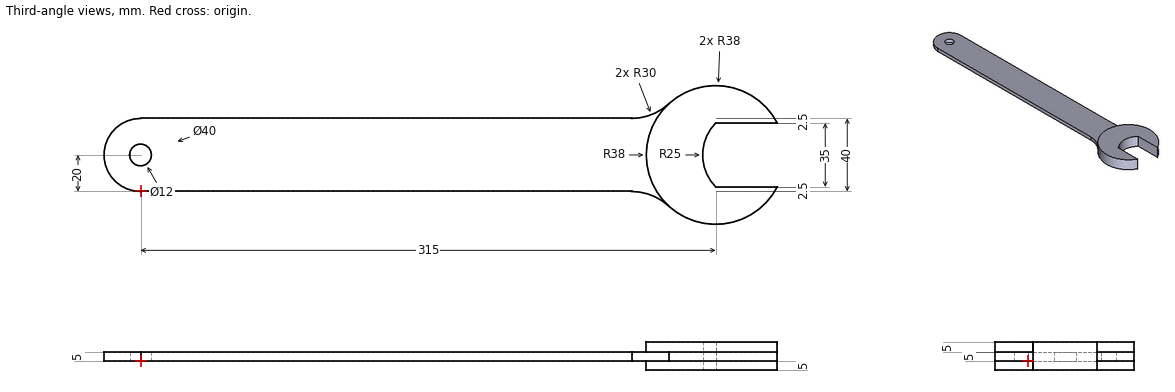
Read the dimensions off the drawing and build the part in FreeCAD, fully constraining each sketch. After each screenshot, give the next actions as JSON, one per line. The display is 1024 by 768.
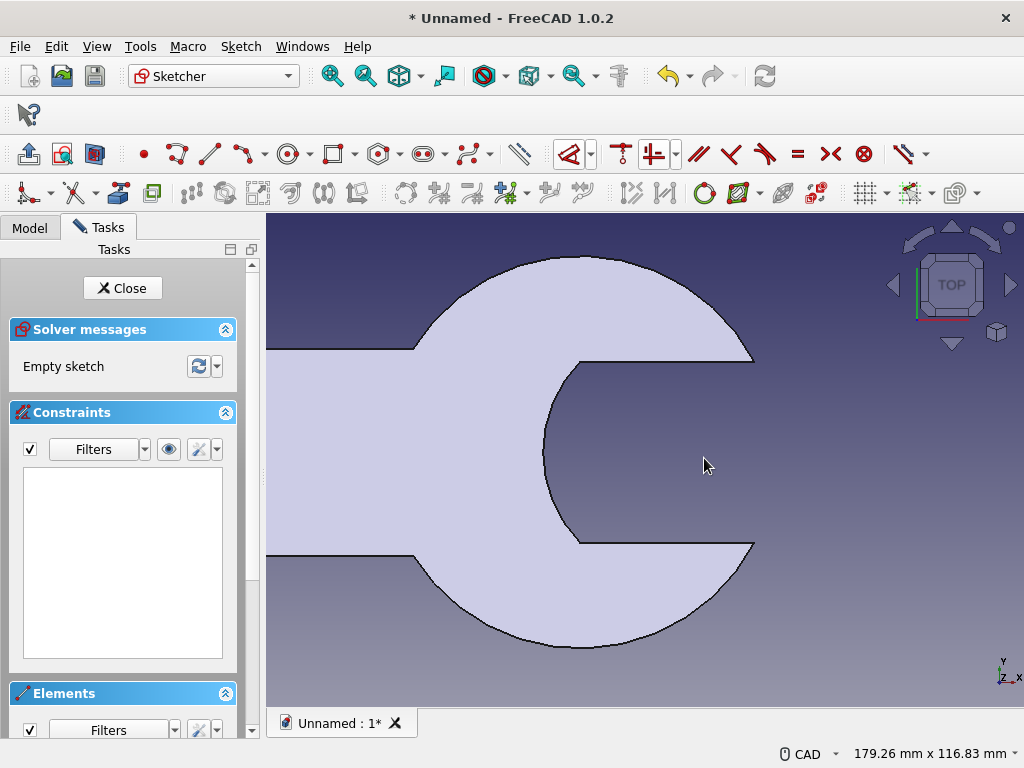
{"action": "left_click", "coordinate": [210, 154]}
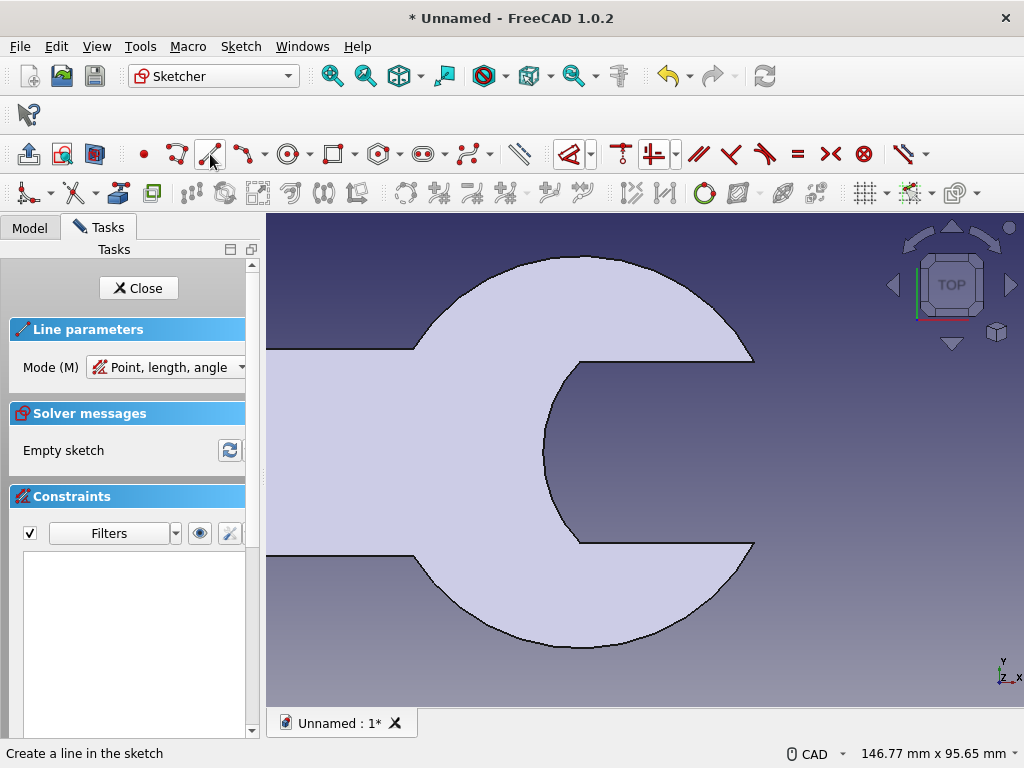
{"action": "left_click", "coordinate": [754, 362]}
{"action": "left_click", "coordinate": [580, 362]}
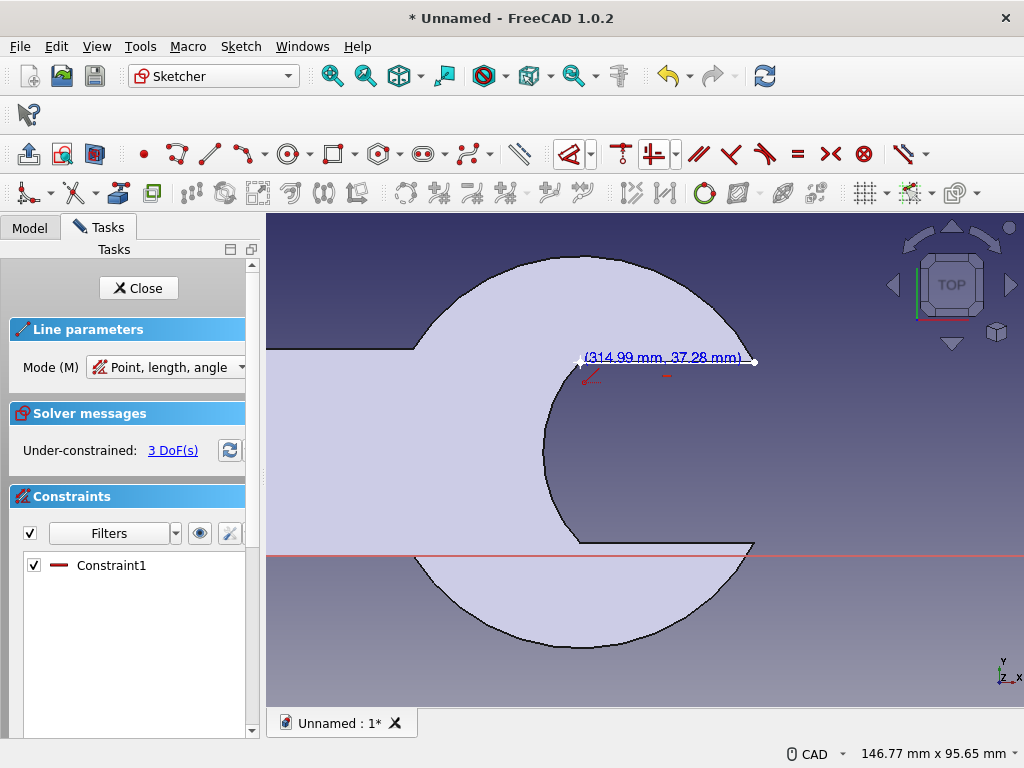
{"action": "scroll", "coordinate": [580, 543], "scroll_direction": "up", "scroll_amount": 2}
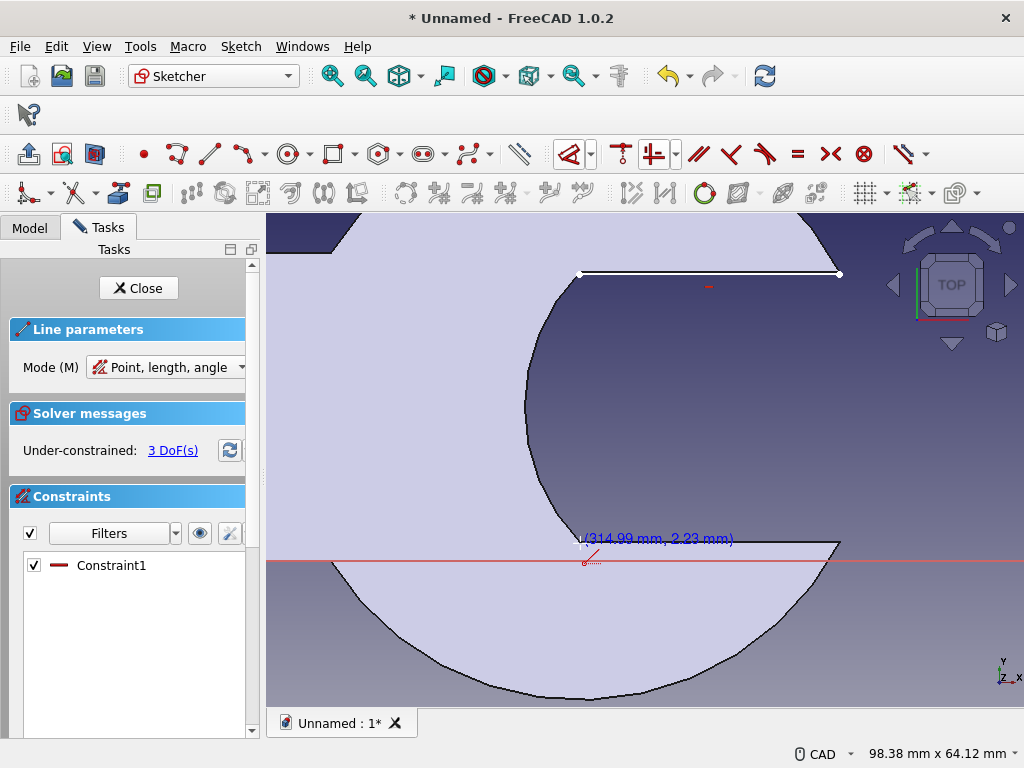
{"action": "left_click", "coordinate": [580, 542]}
{"action": "left_click", "coordinate": [840, 542]}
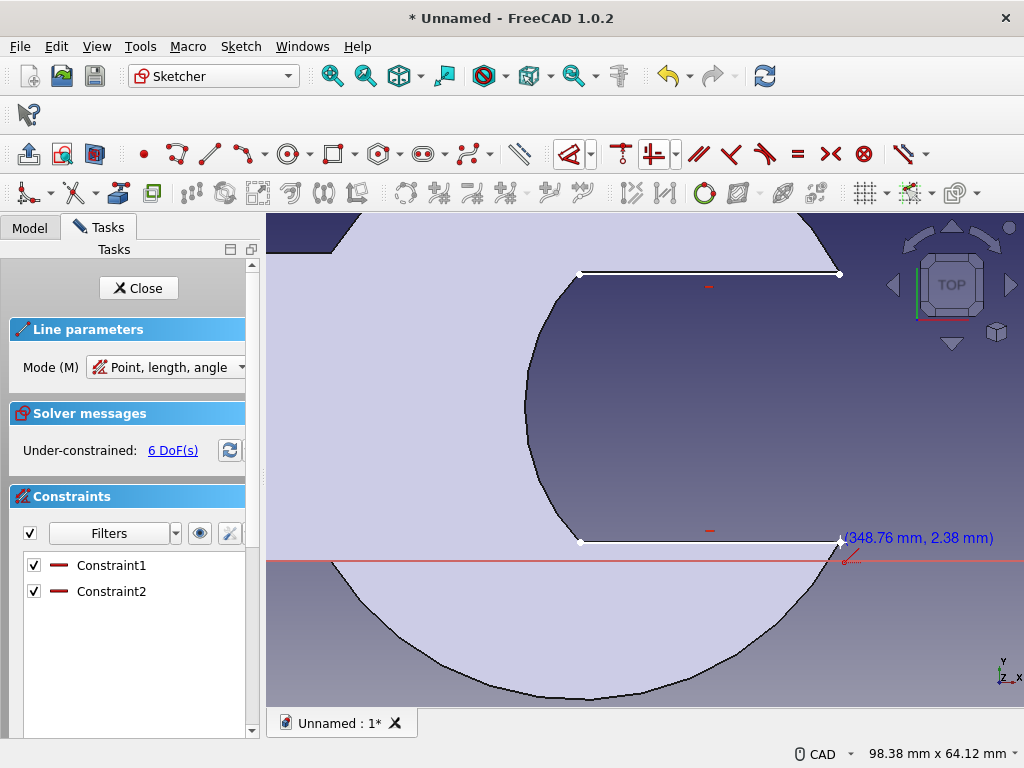
{"action": "left_click", "coordinate": [242, 154]}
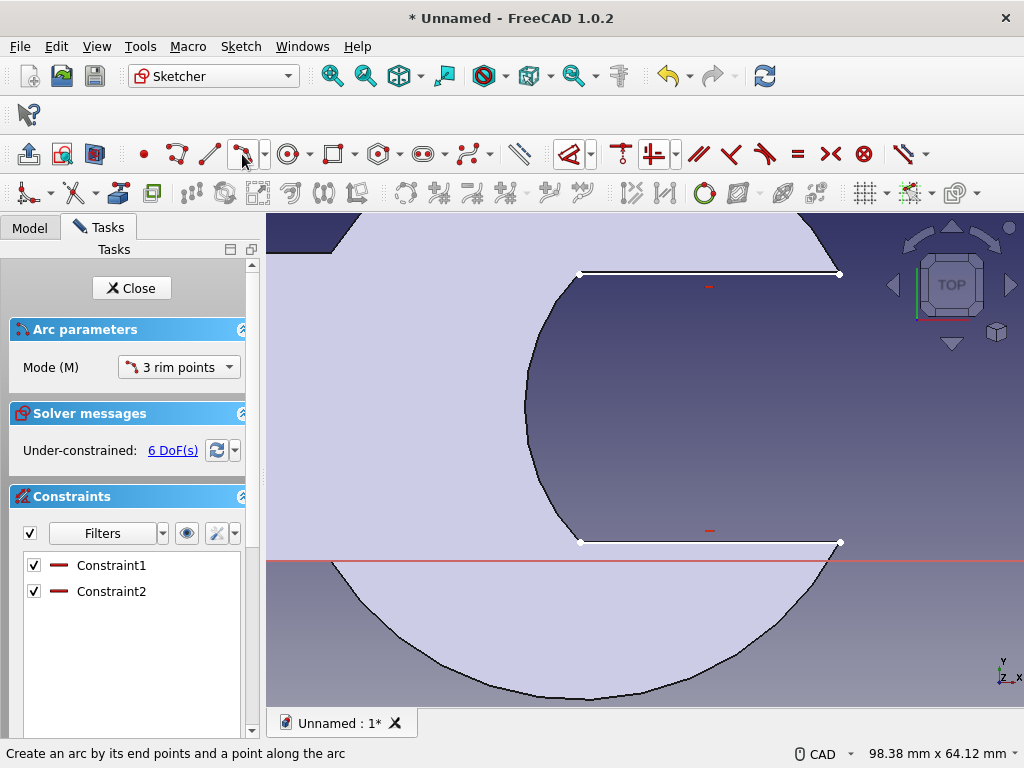
{"action": "left_click", "coordinate": [580, 274]}
{"action": "left_click", "coordinate": [580, 543]}
{"action": "left_click", "coordinate": [525, 407]}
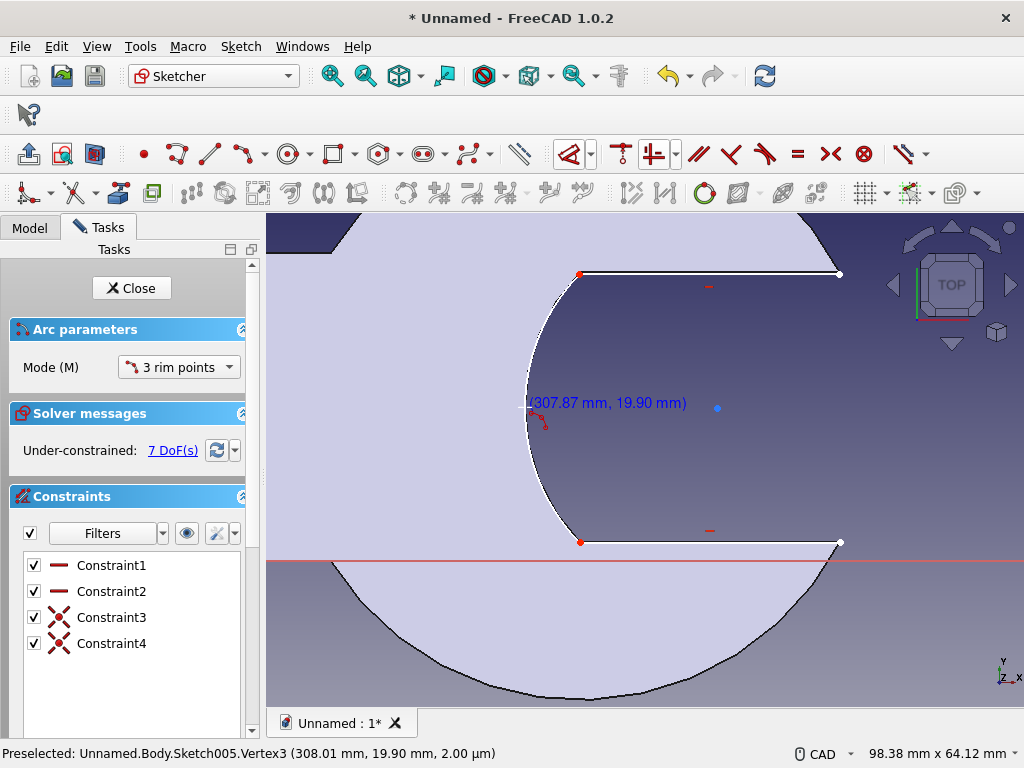
{"action": "left_click", "coordinate": [840, 543]}
{"action": "left_click", "coordinate": [839, 274]}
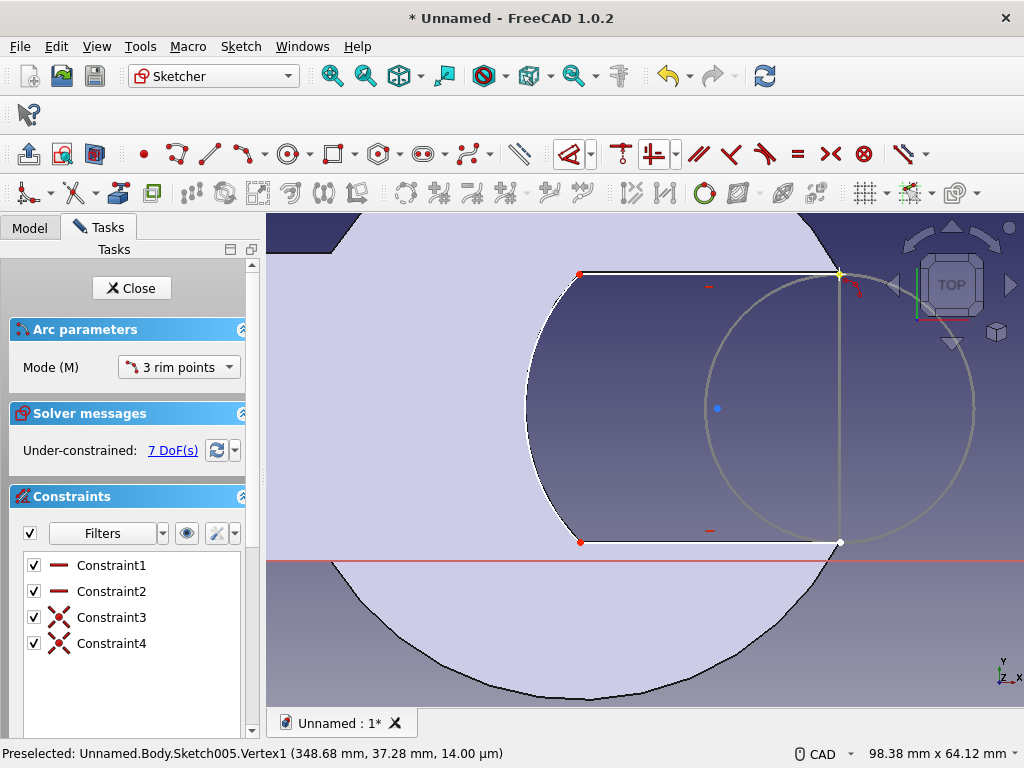
{"action": "scroll", "coordinate": [603, 567], "scroll_direction": "down", "scroll_amount": 2}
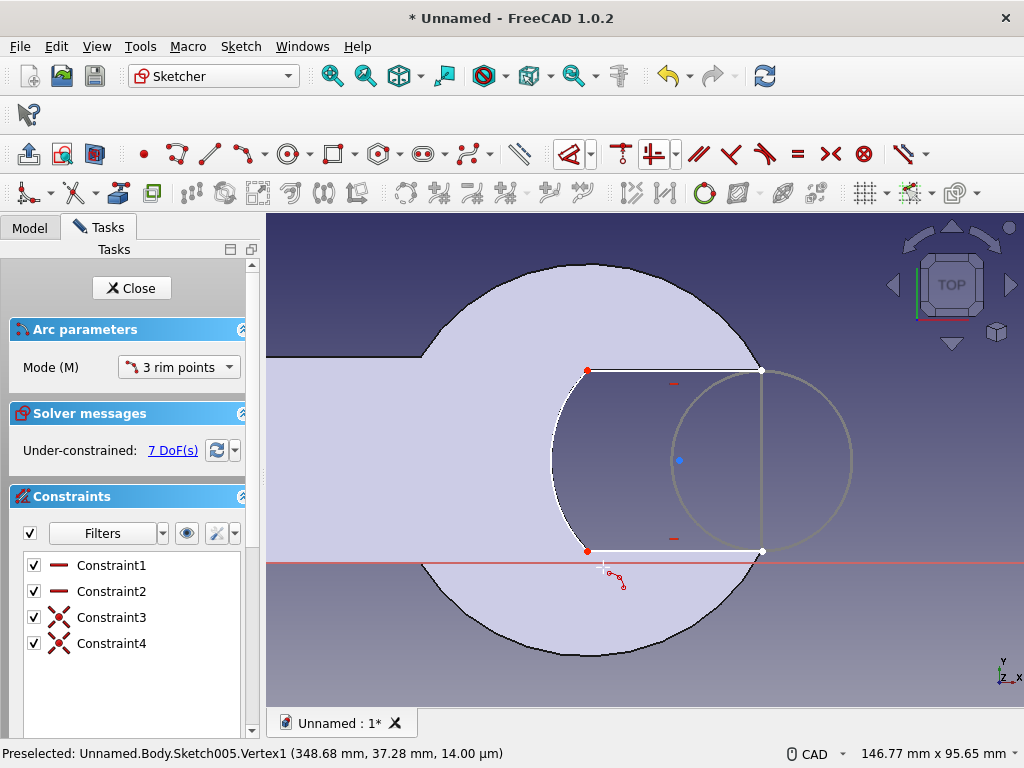
{"action": "left_click", "coordinate": [391, 460]}
{"action": "key", "text": "Escape"}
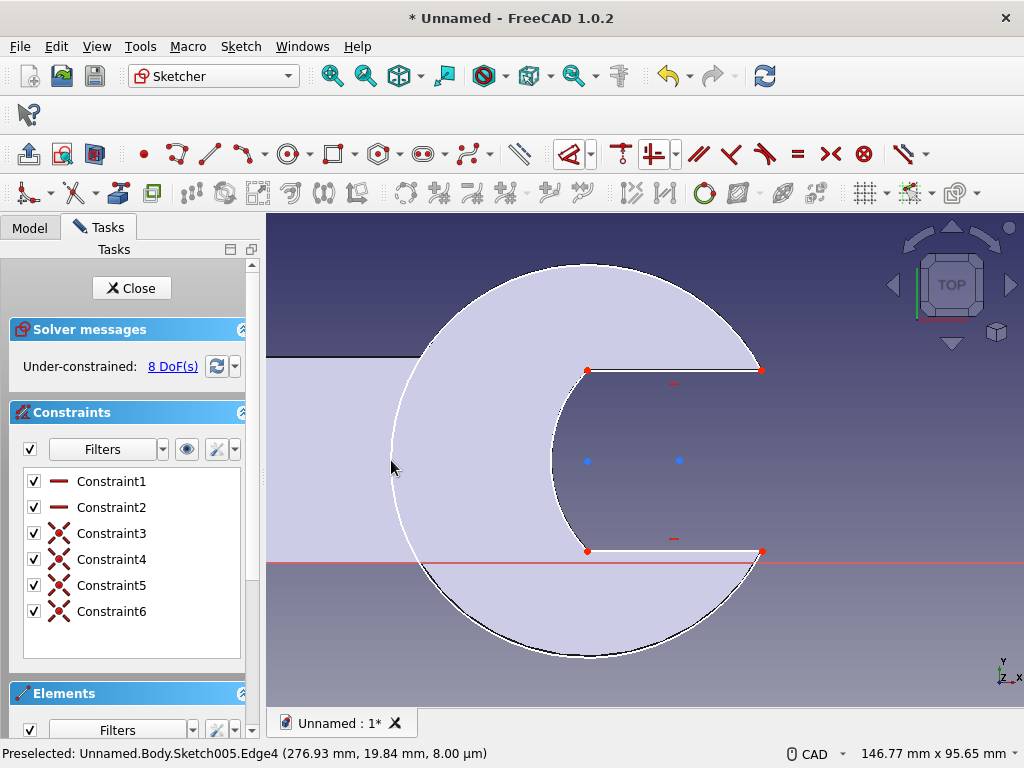
{"action": "left_click", "coordinate": [557, 422]}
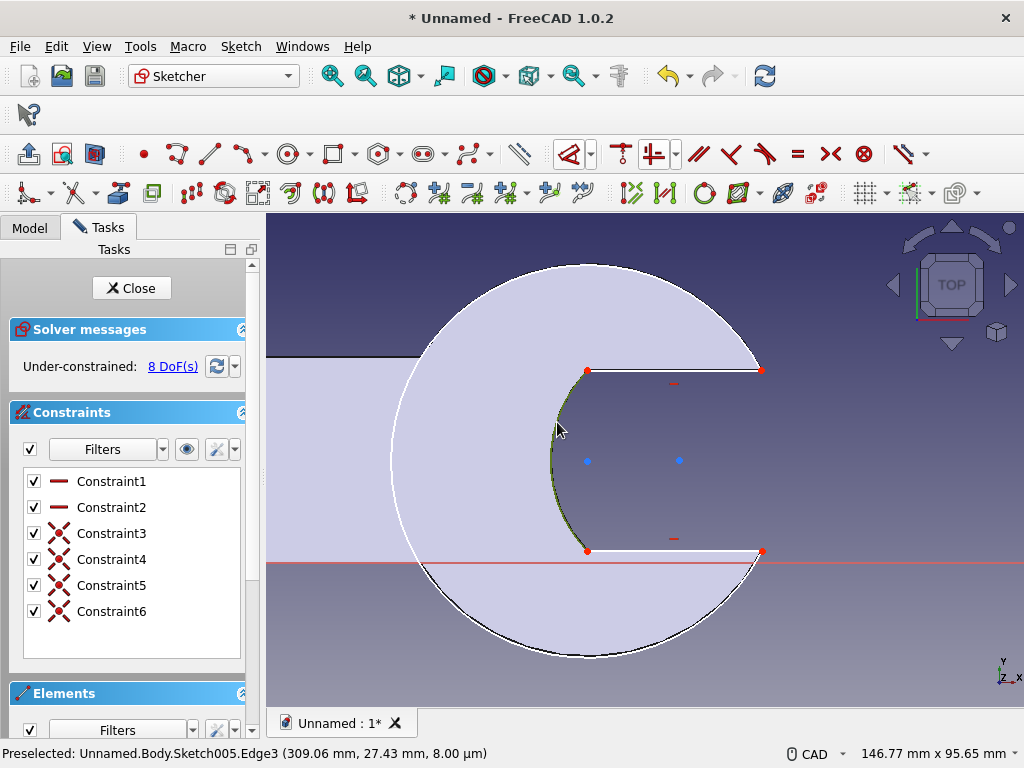
{"action": "left_click", "coordinate": [590, 154]}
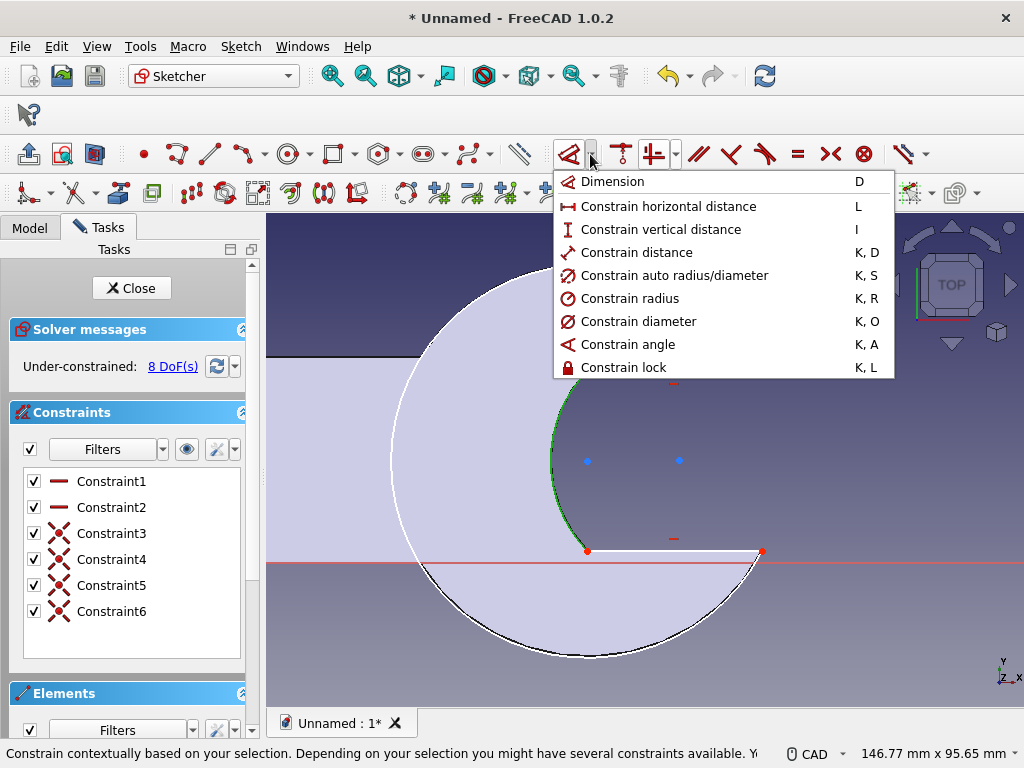
{"action": "left_click", "coordinate": [724, 298]}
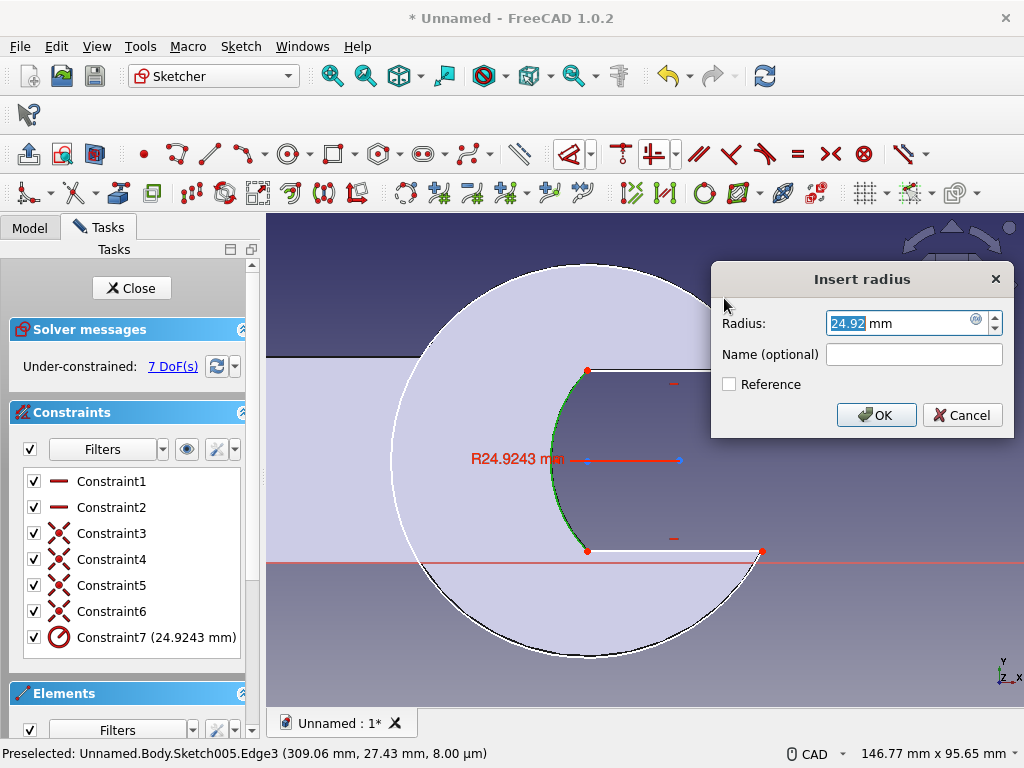
{"action": "type", "text": "25"}
{"action": "key", "text": "Return"}